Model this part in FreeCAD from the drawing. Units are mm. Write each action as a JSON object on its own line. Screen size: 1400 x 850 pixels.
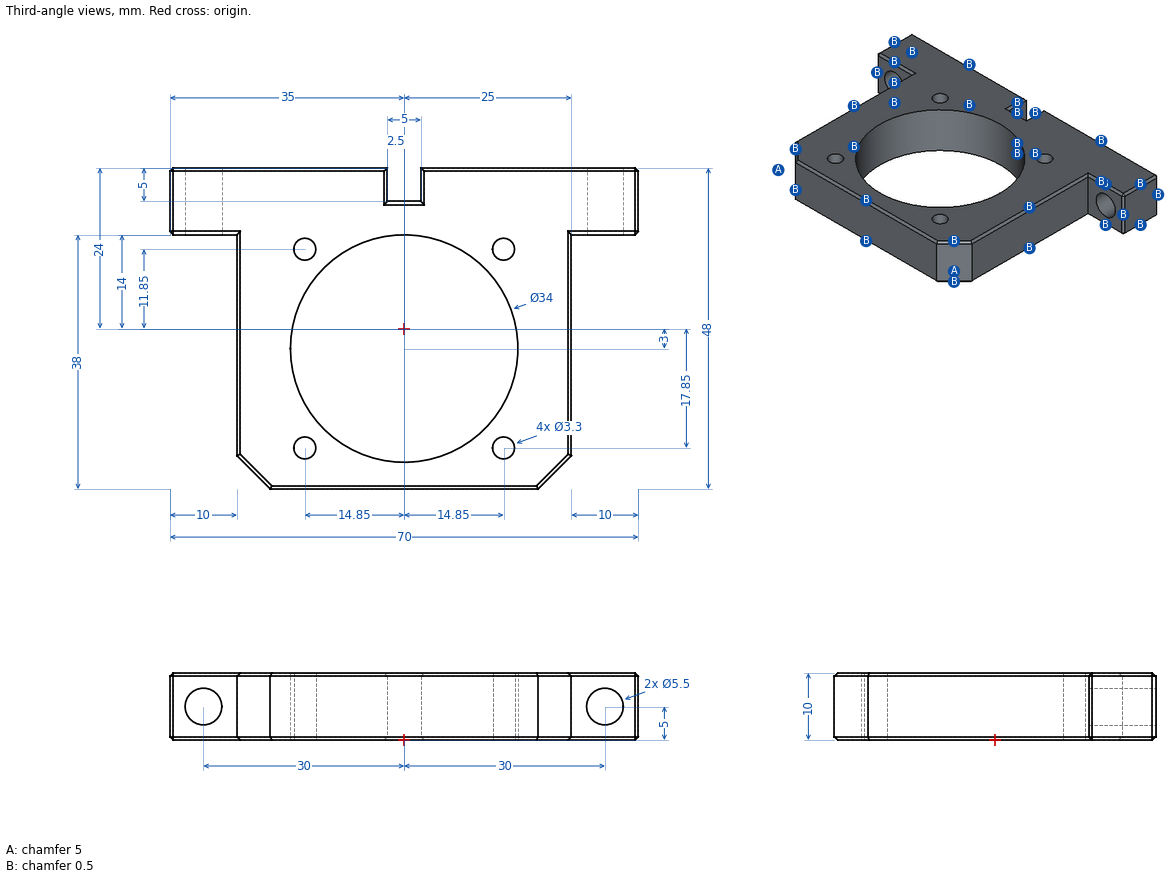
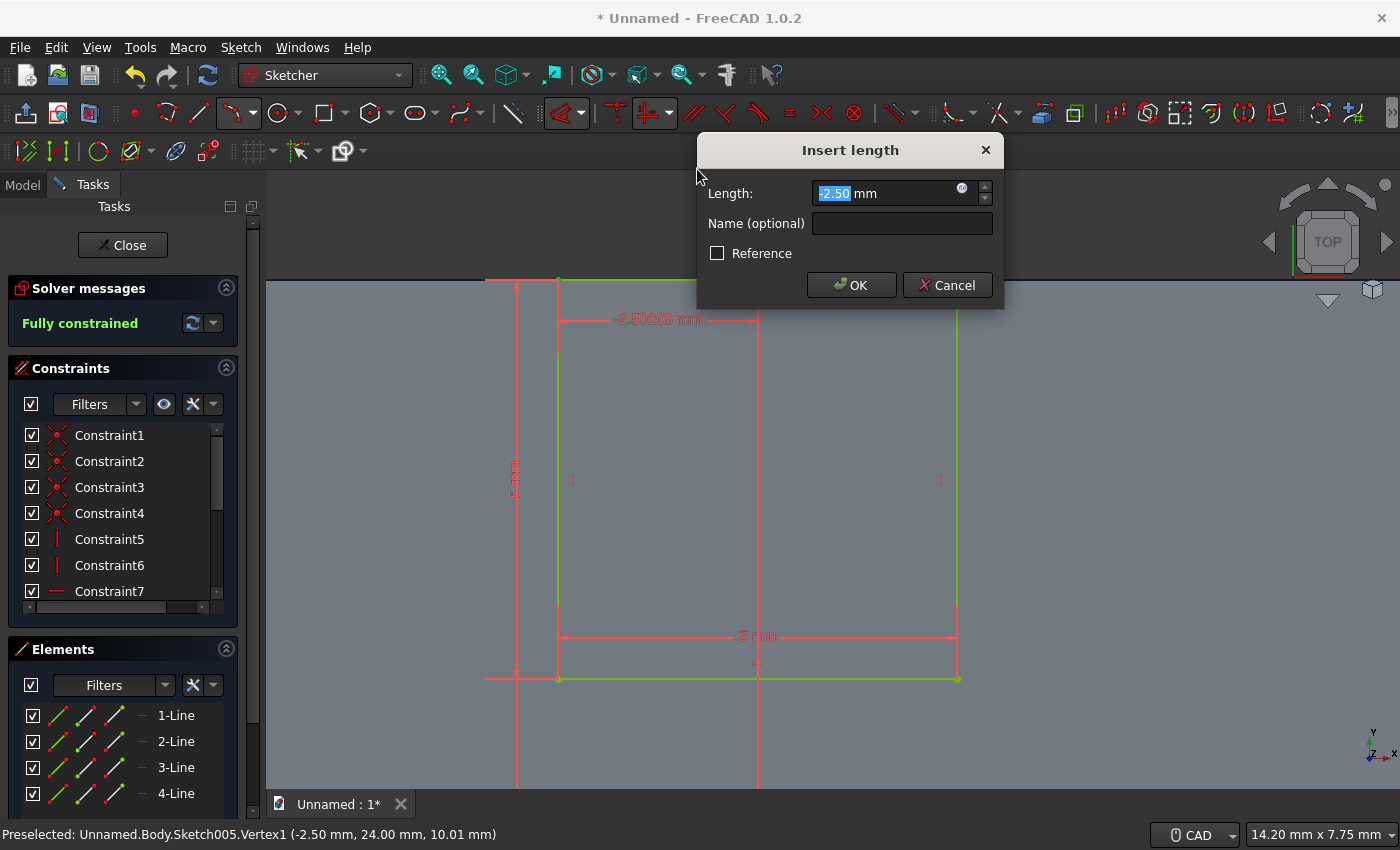
{"action": "type", "text": "-2.5"}
{"action": "key", "text": "Return"}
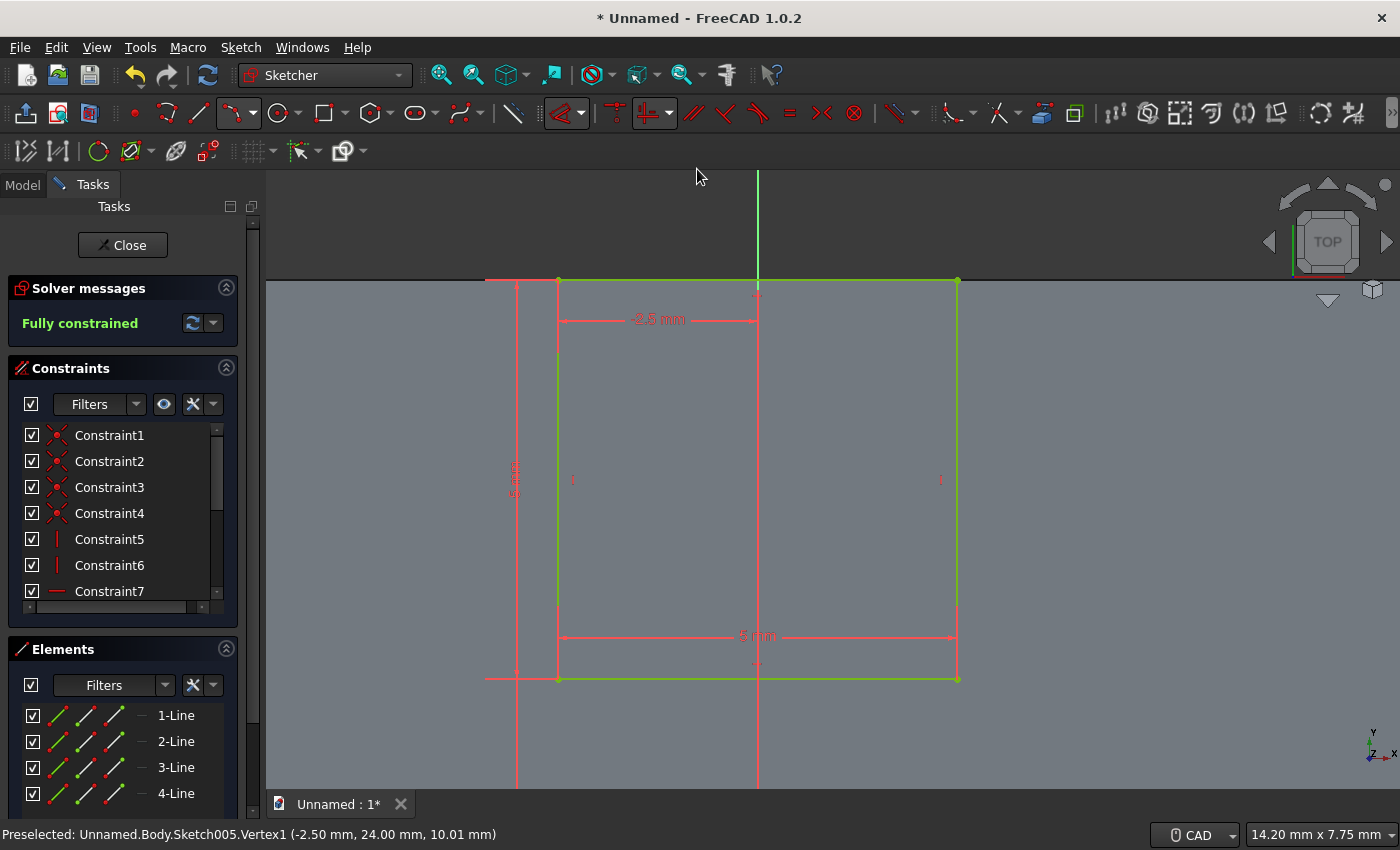
{"action": "left_click", "coordinate": [123, 245]}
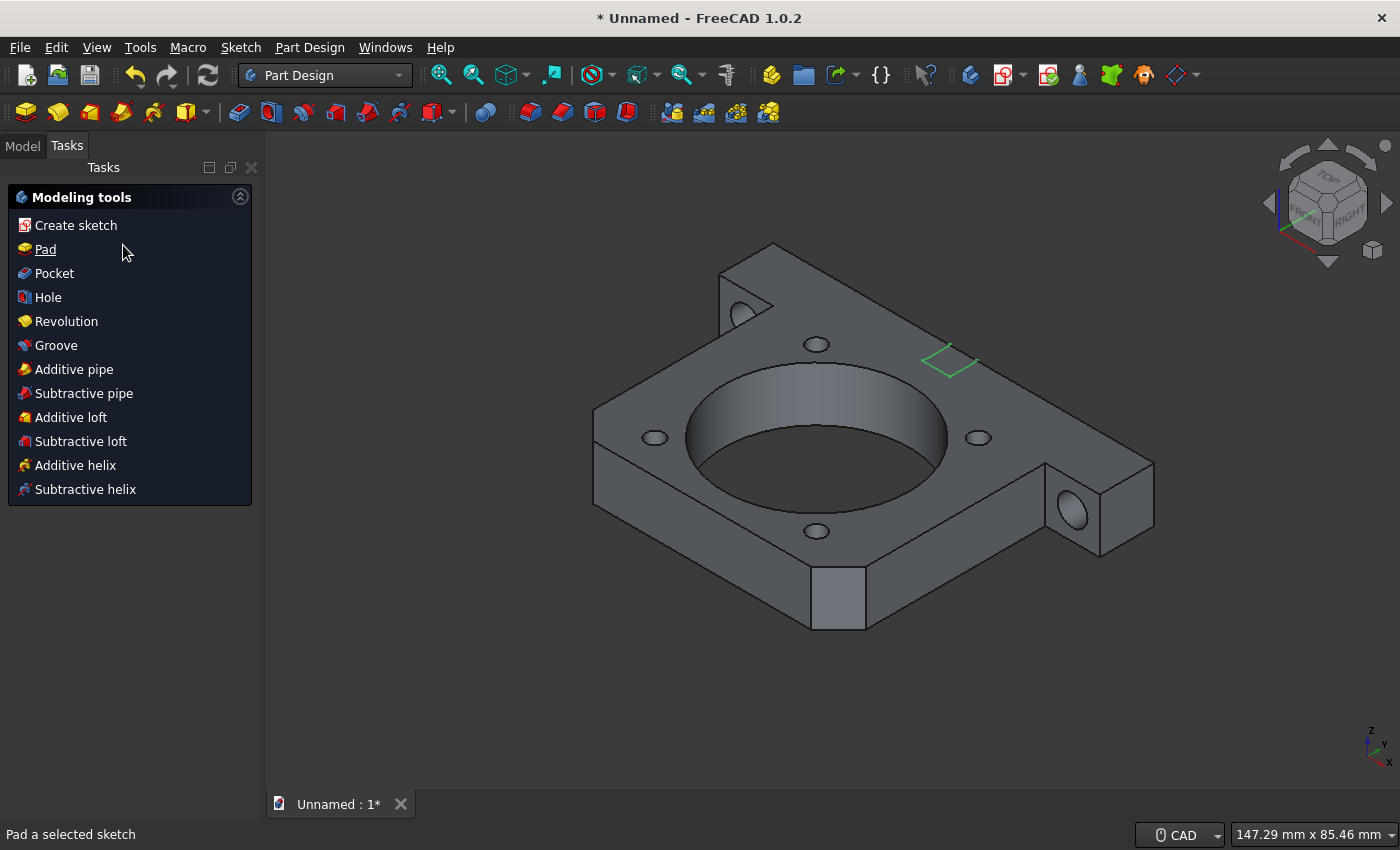
{"action": "left_click", "coordinate": [240, 112]}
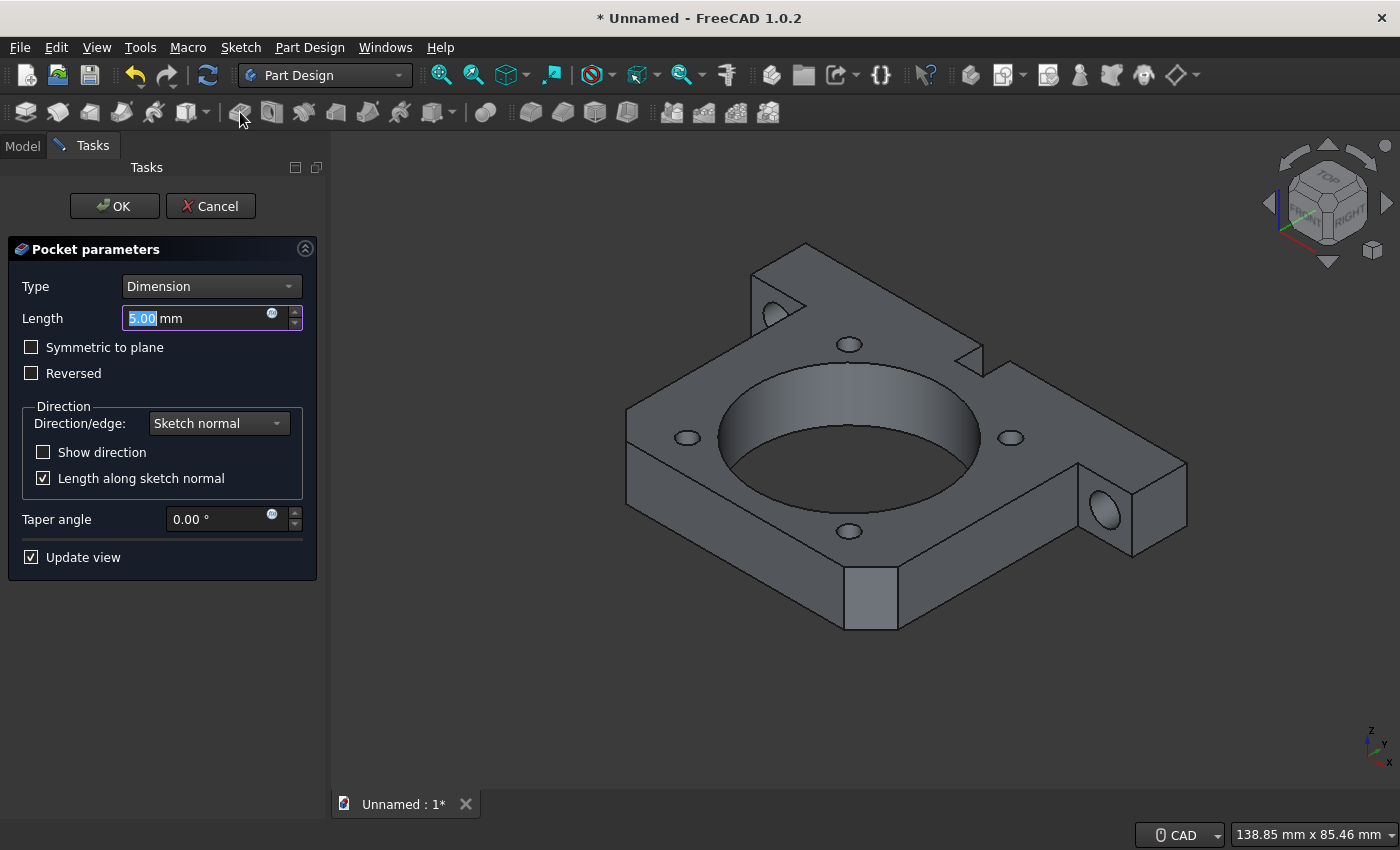
{"action": "left_click", "coordinate": [212, 286]}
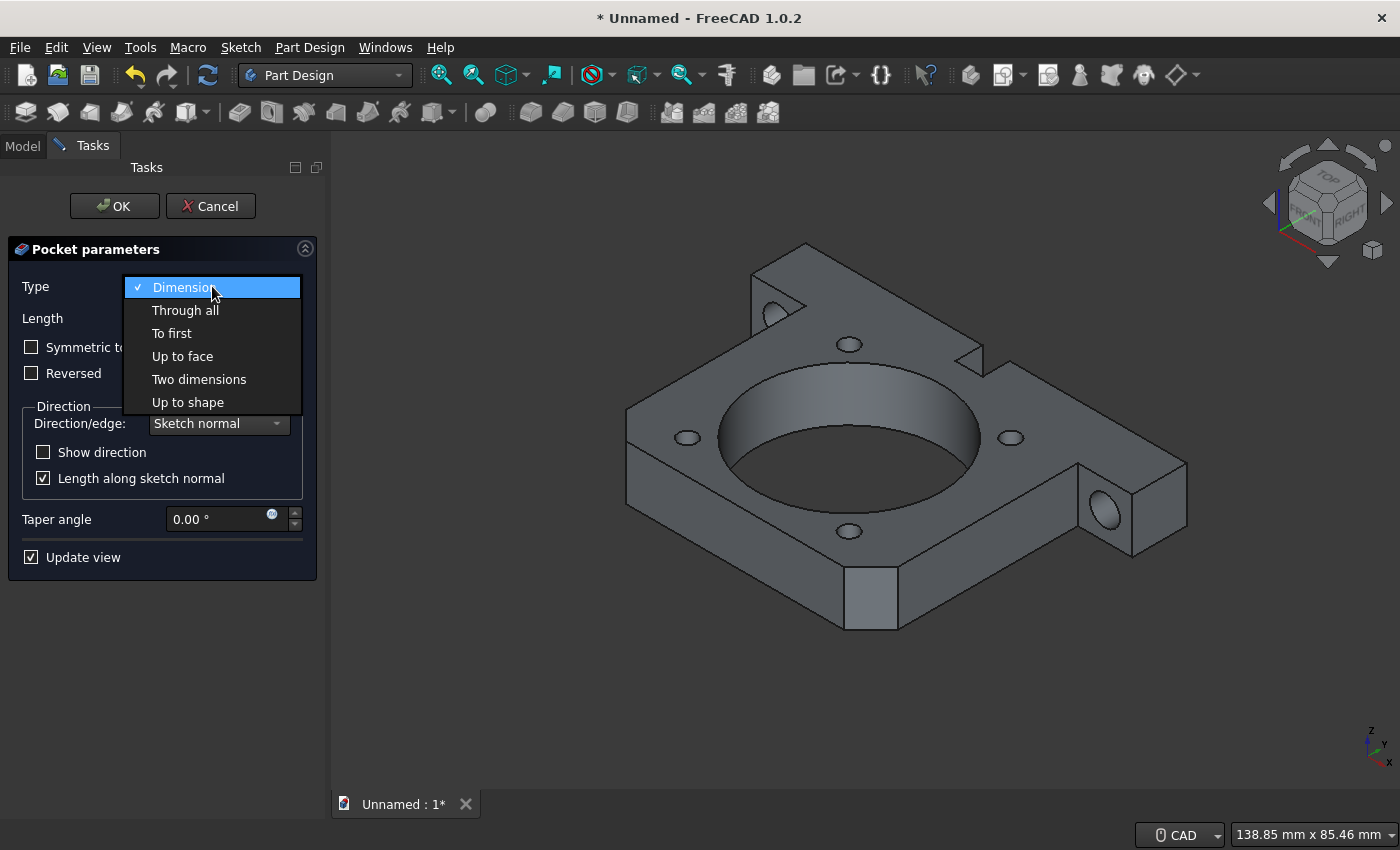
{"action": "left_click", "coordinate": [212, 310]}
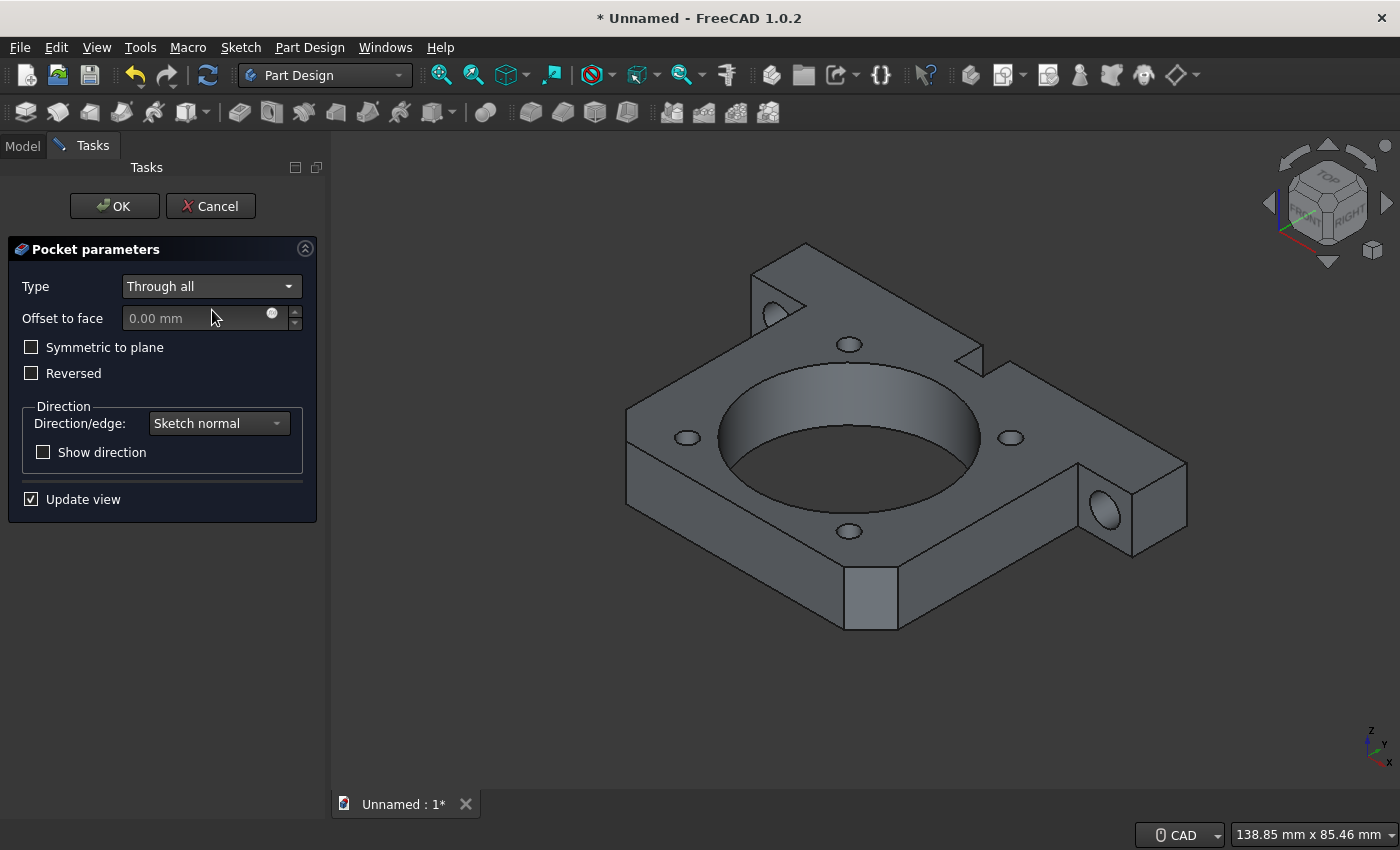
{"action": "left_click", "coordinate": [115, 206]}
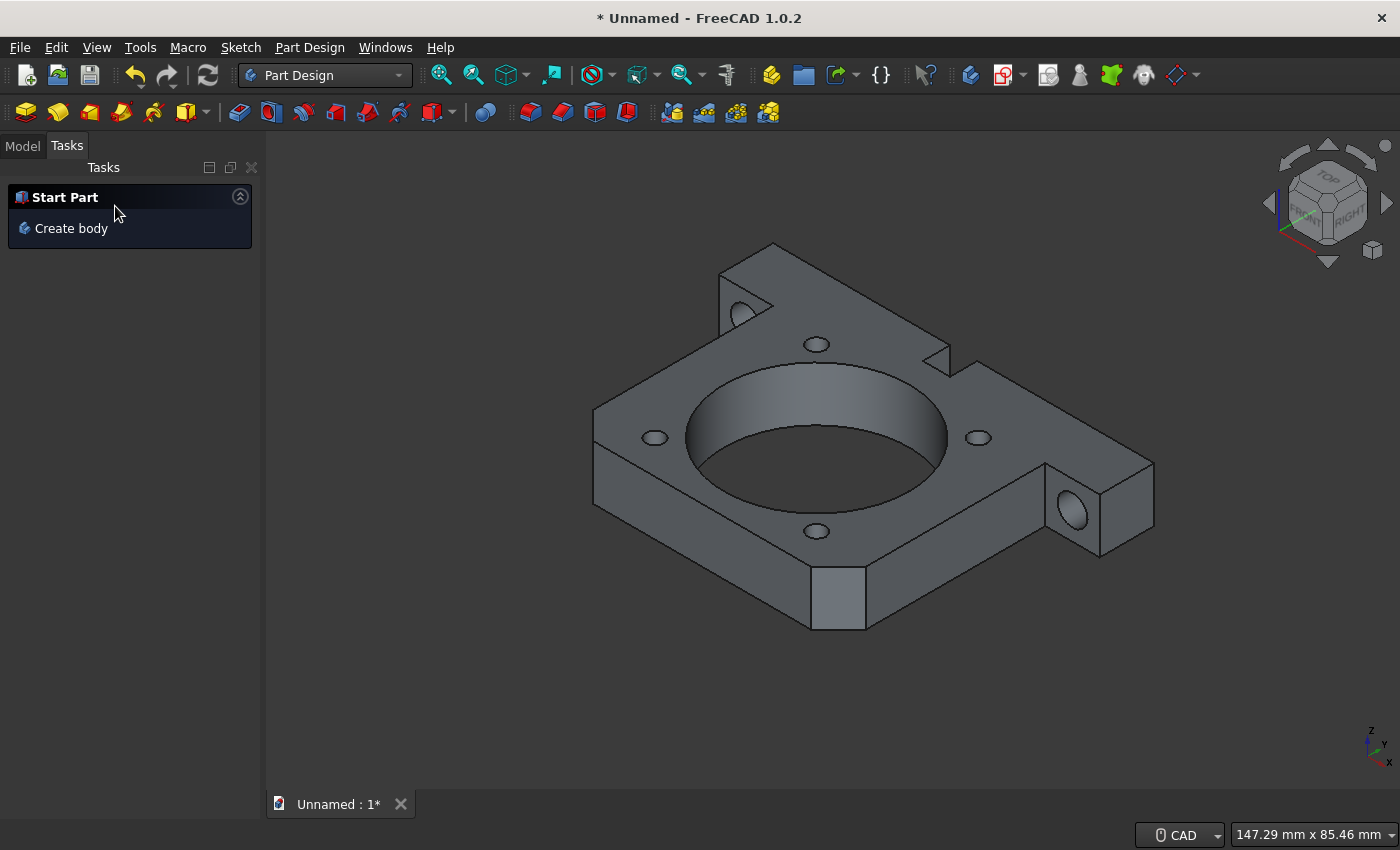
{"action": "left_click", "coordinate": [1127, 509]}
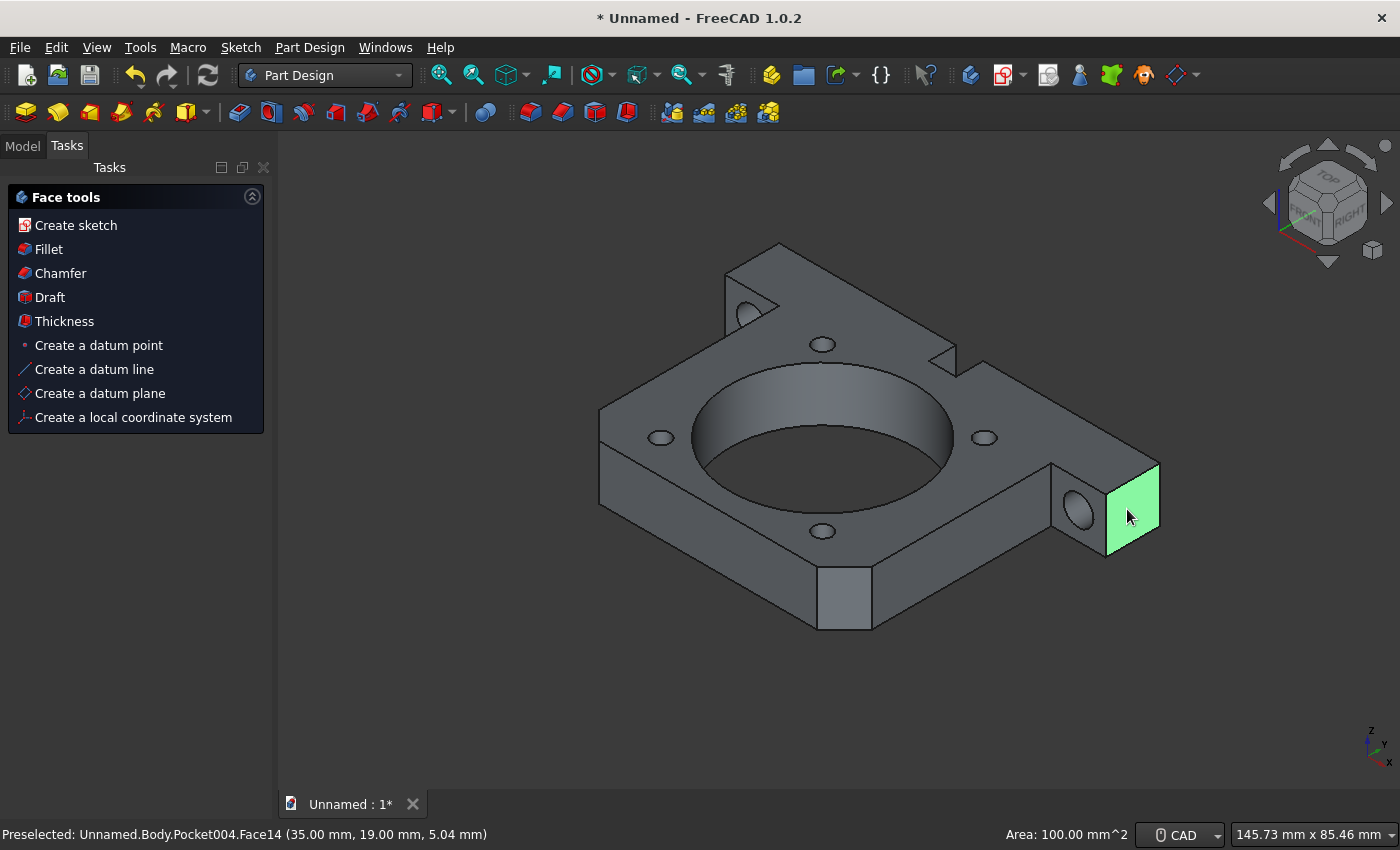
{"action": "left_click", "coordinate": [752, 289], "text": "ctrl"}